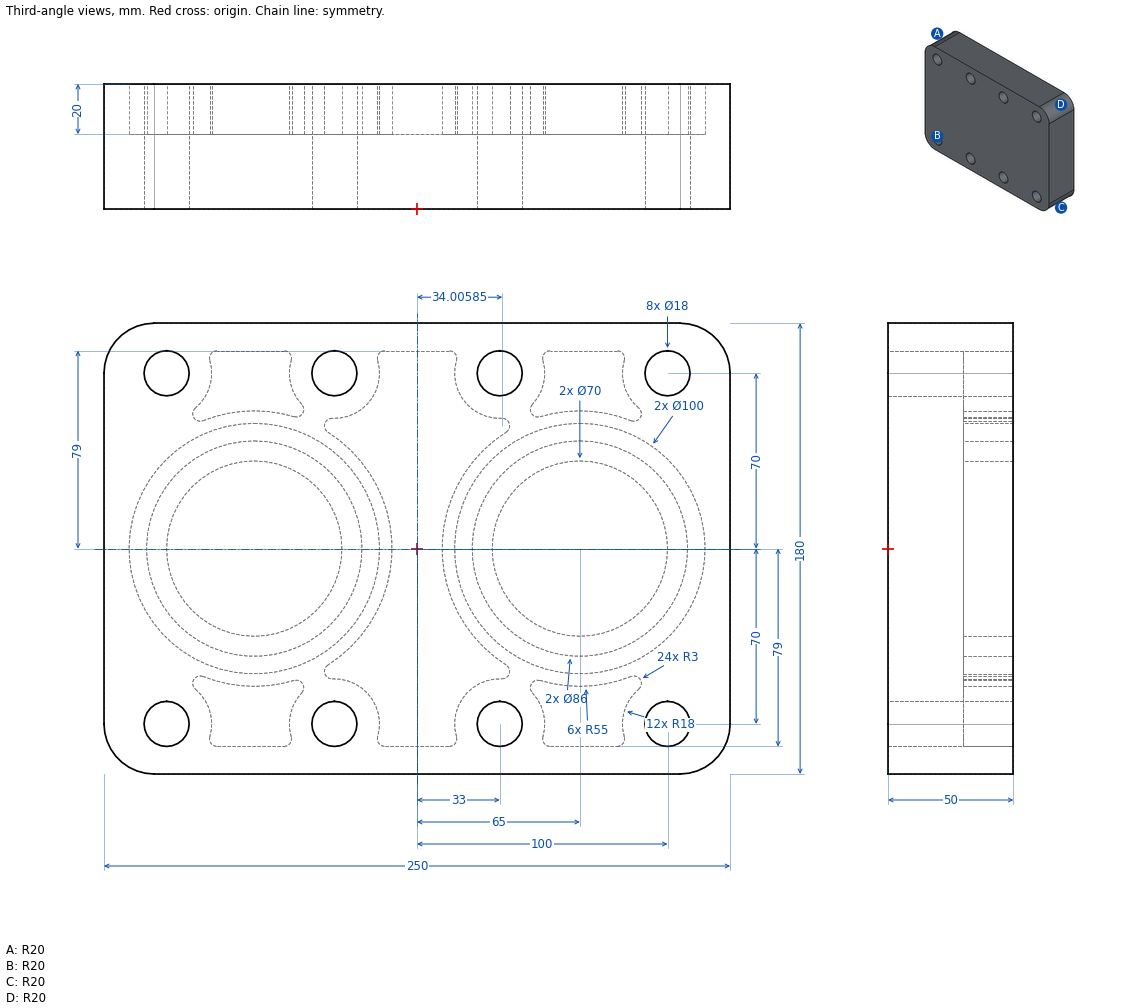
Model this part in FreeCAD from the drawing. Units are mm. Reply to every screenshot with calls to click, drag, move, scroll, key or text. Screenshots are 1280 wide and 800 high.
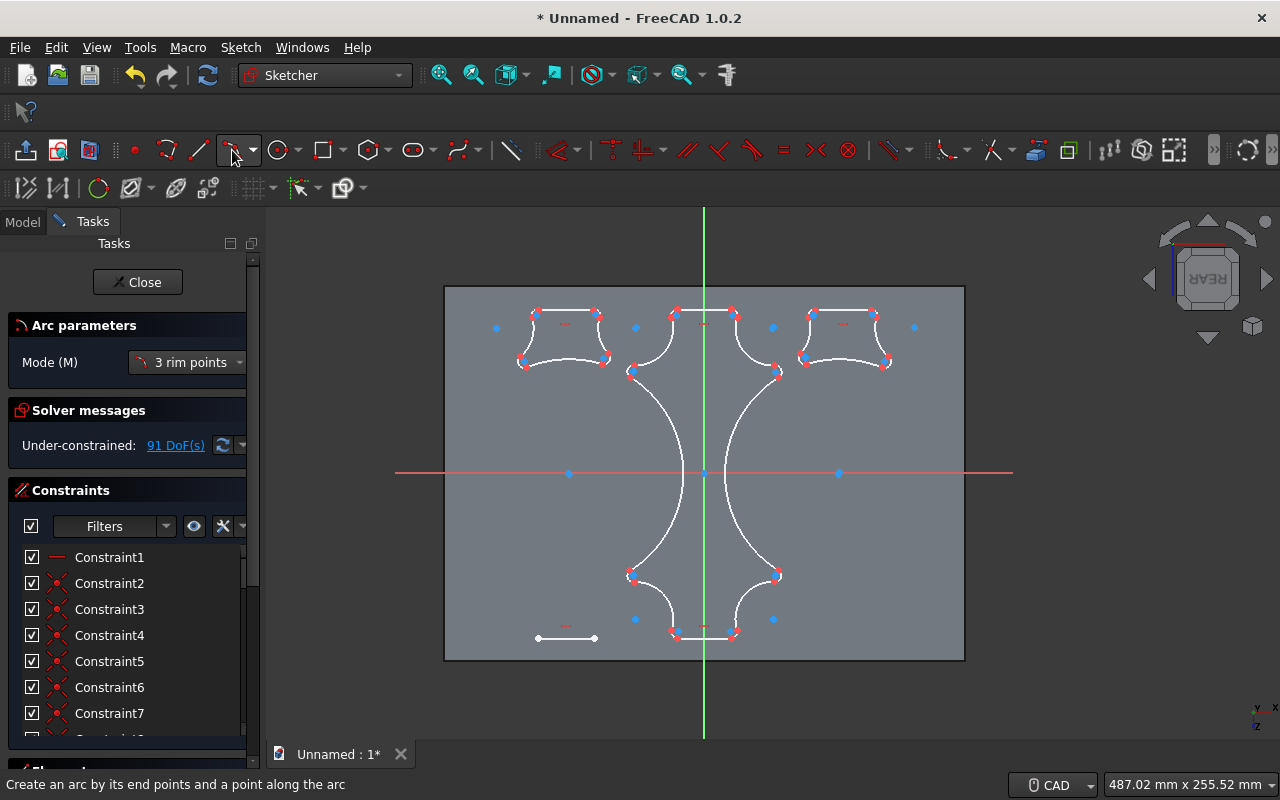
click(594, 639)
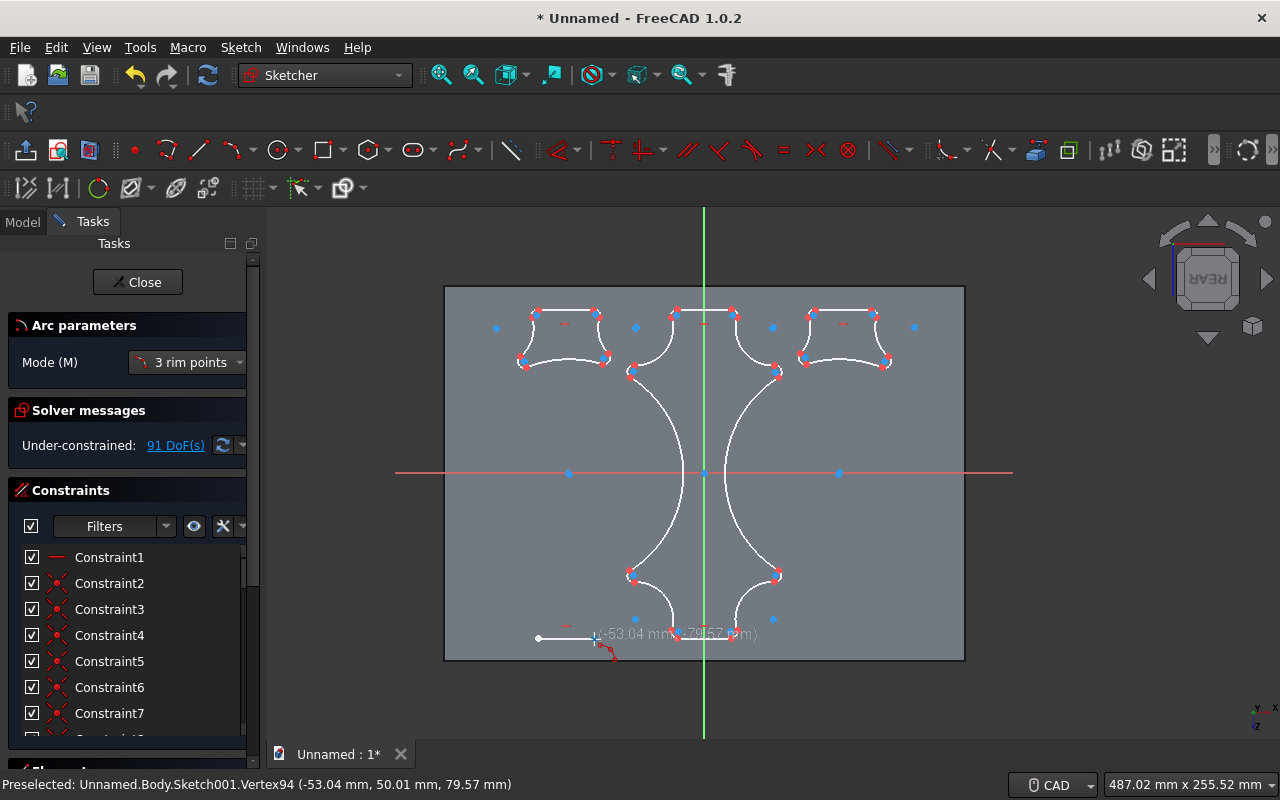
scroll(600, 630, up, 3)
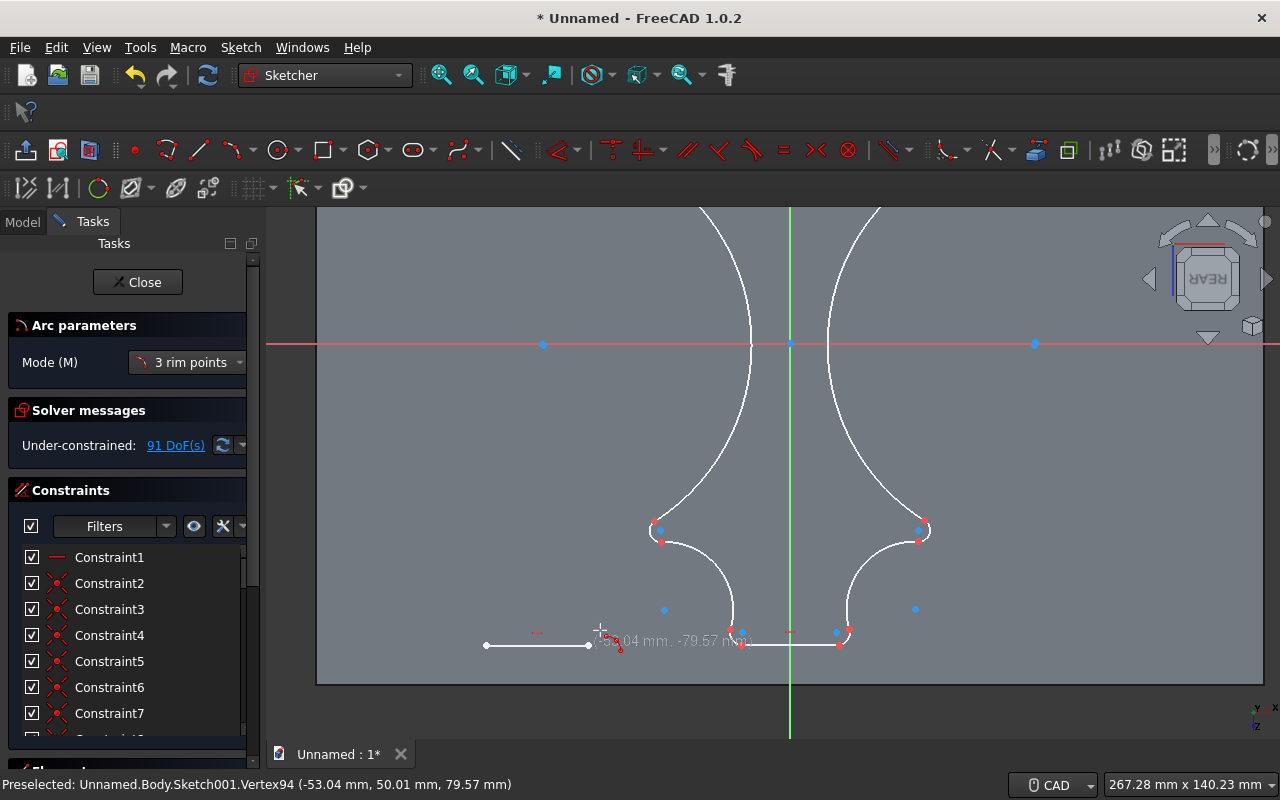
click(599, 629)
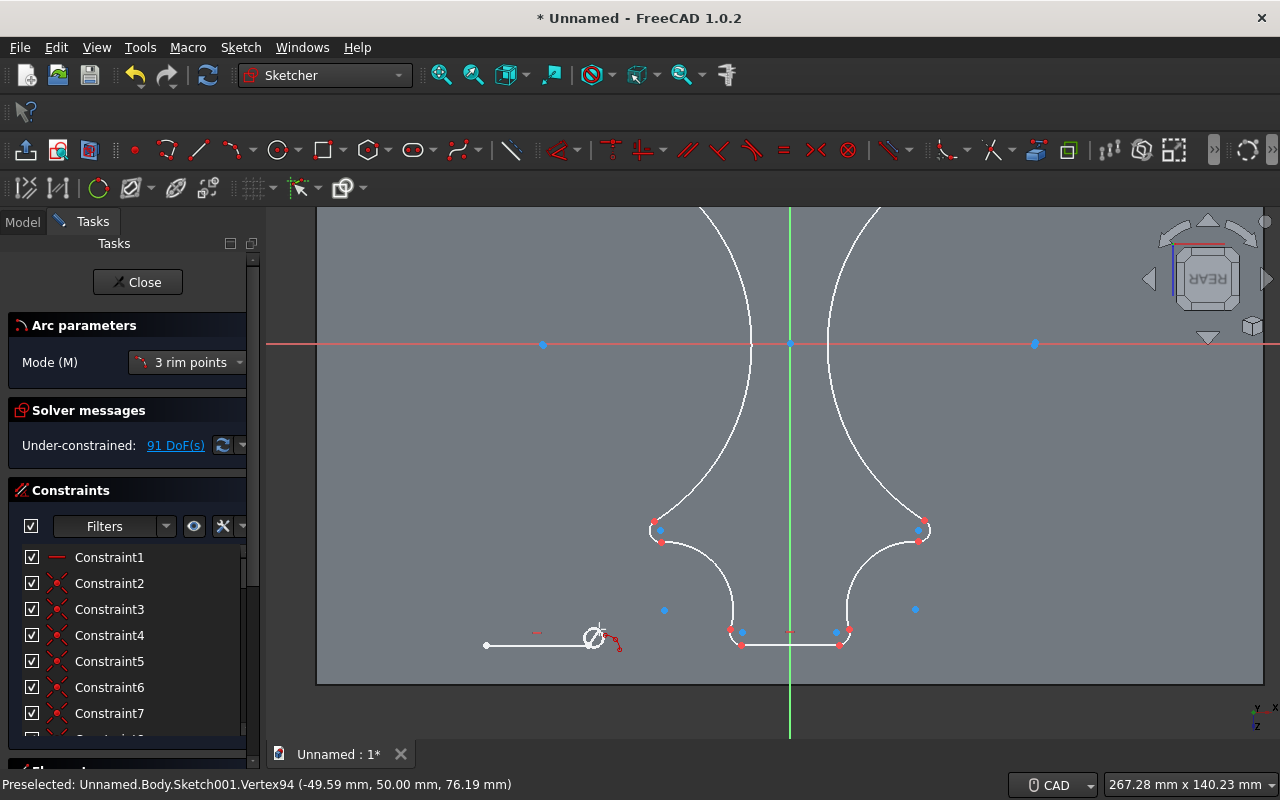
scroll(598, 639, up, 7)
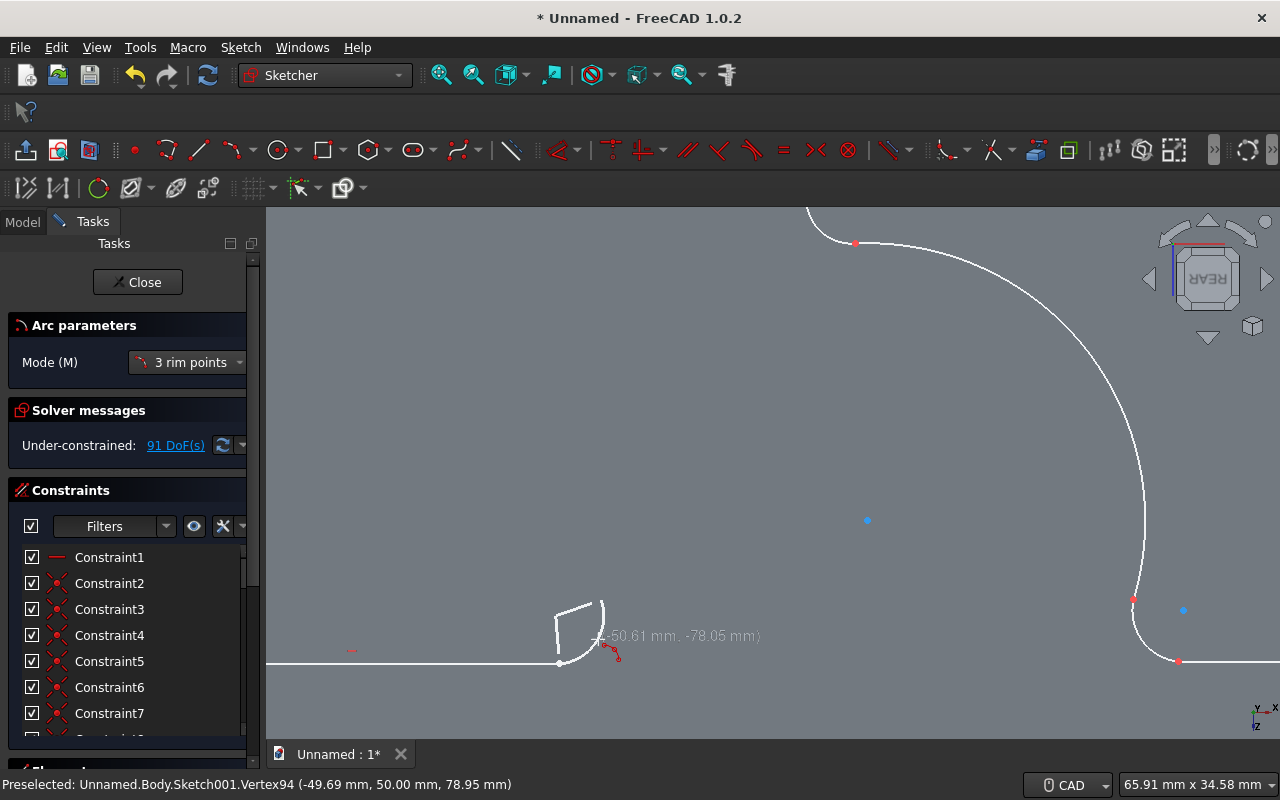
click(595, 637)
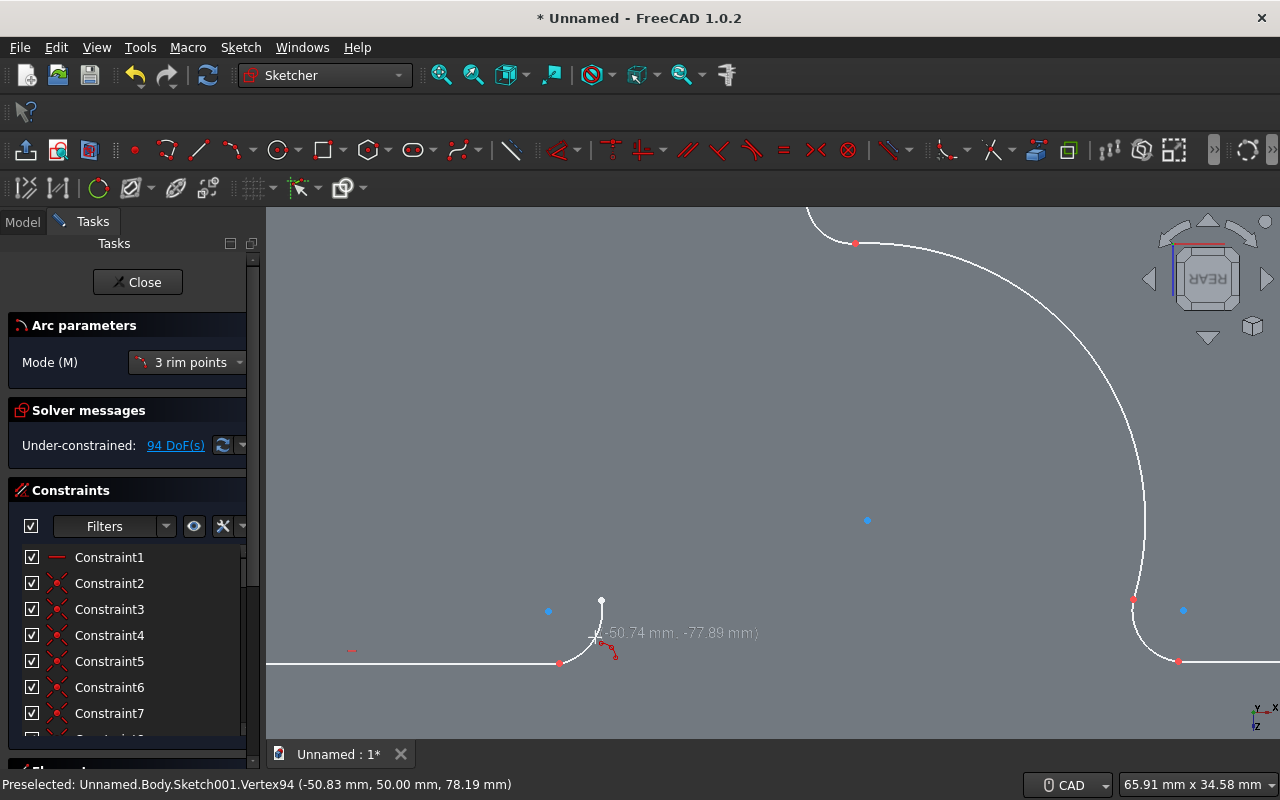
scroll(599, 635, down, 10)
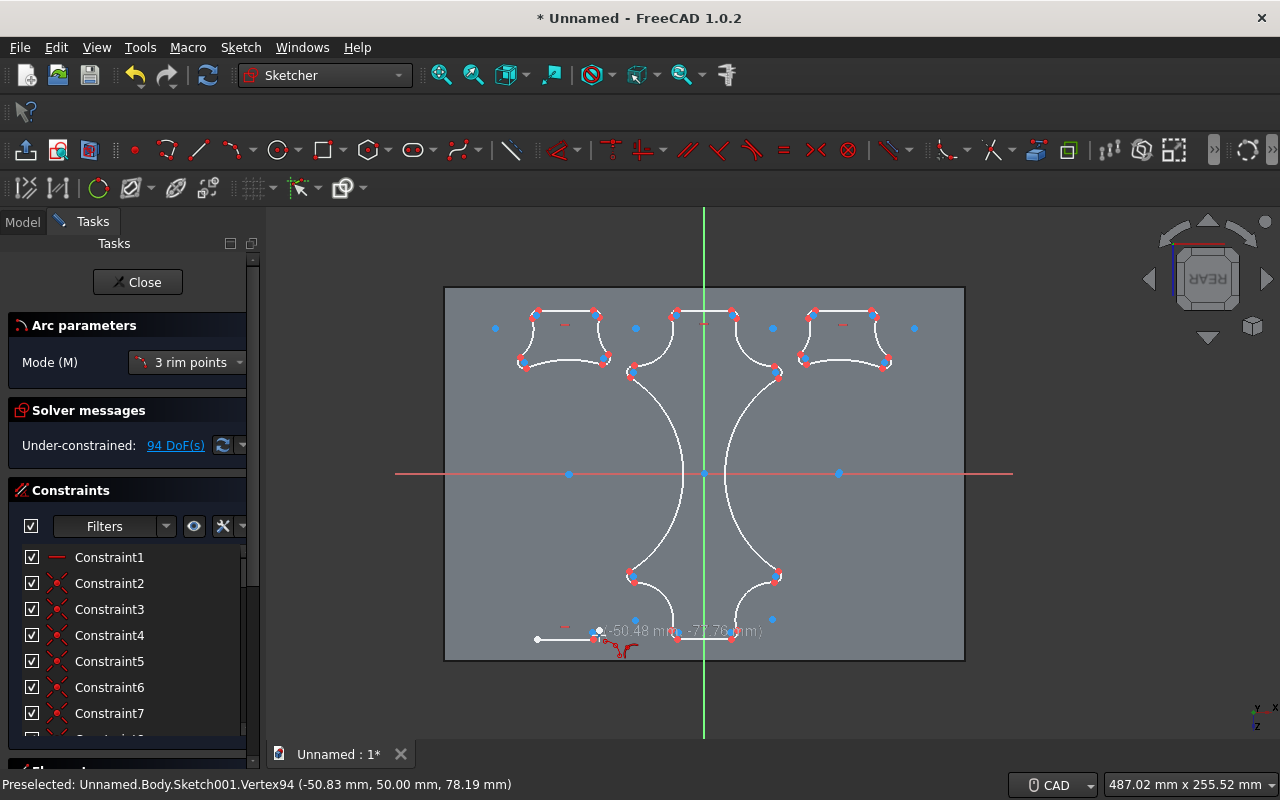
scroll(600, 630, up, 5)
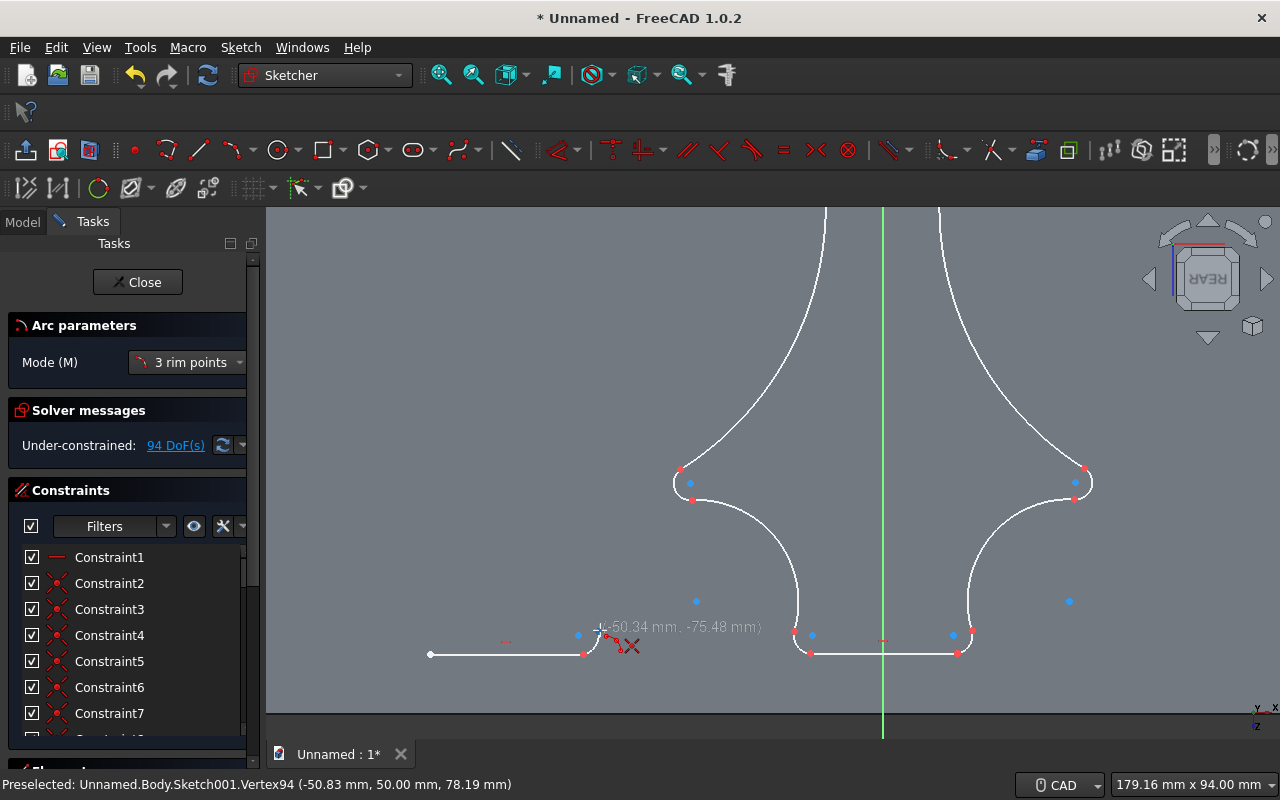
click(598, 631)
click(623, 530)
click(597, 577)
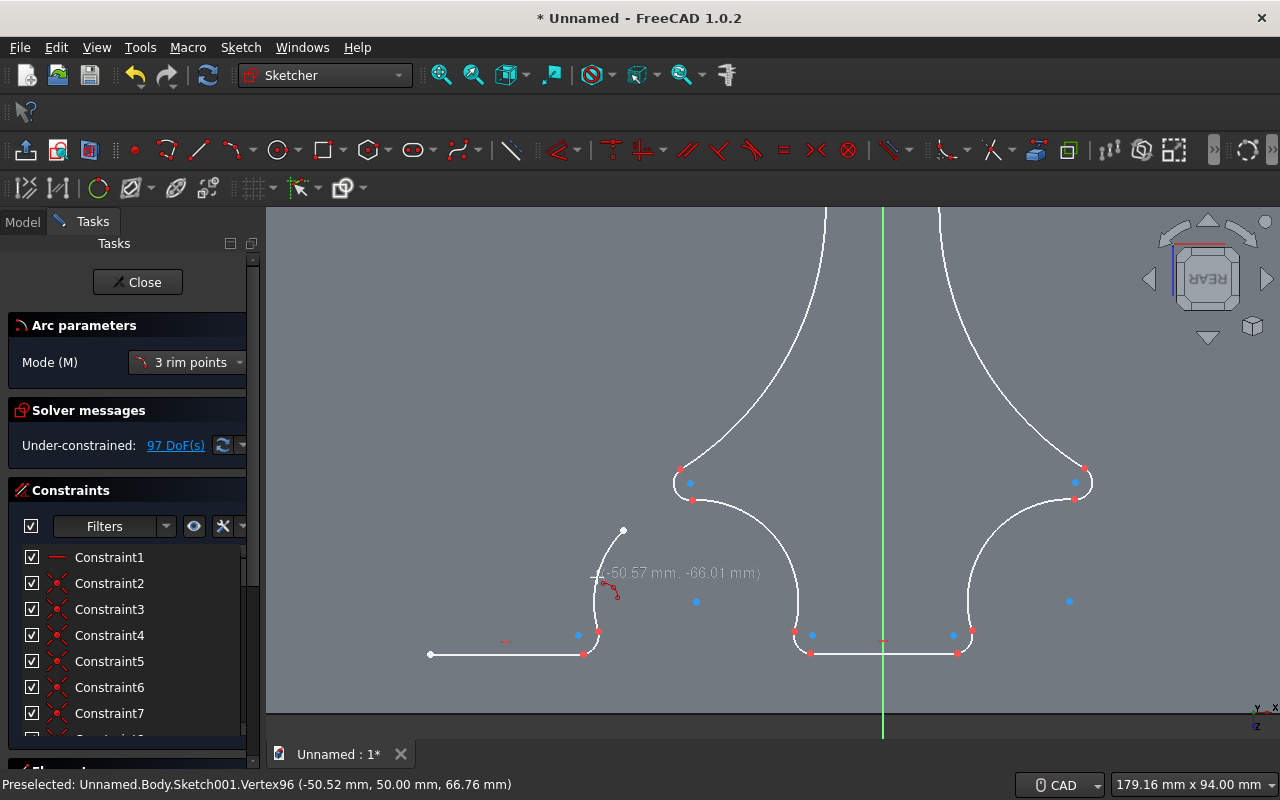
click(623, 531)
click(605, 502)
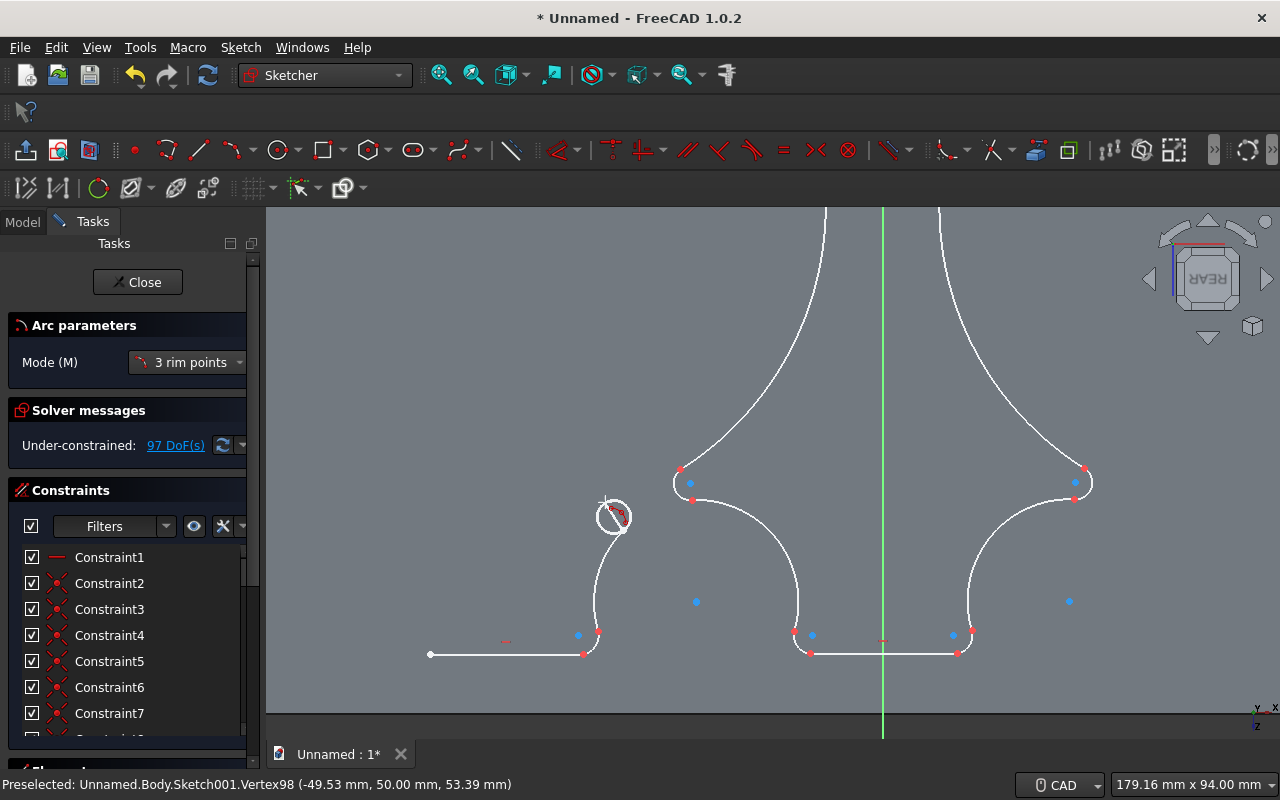
scroll(625, 510, up, 2)